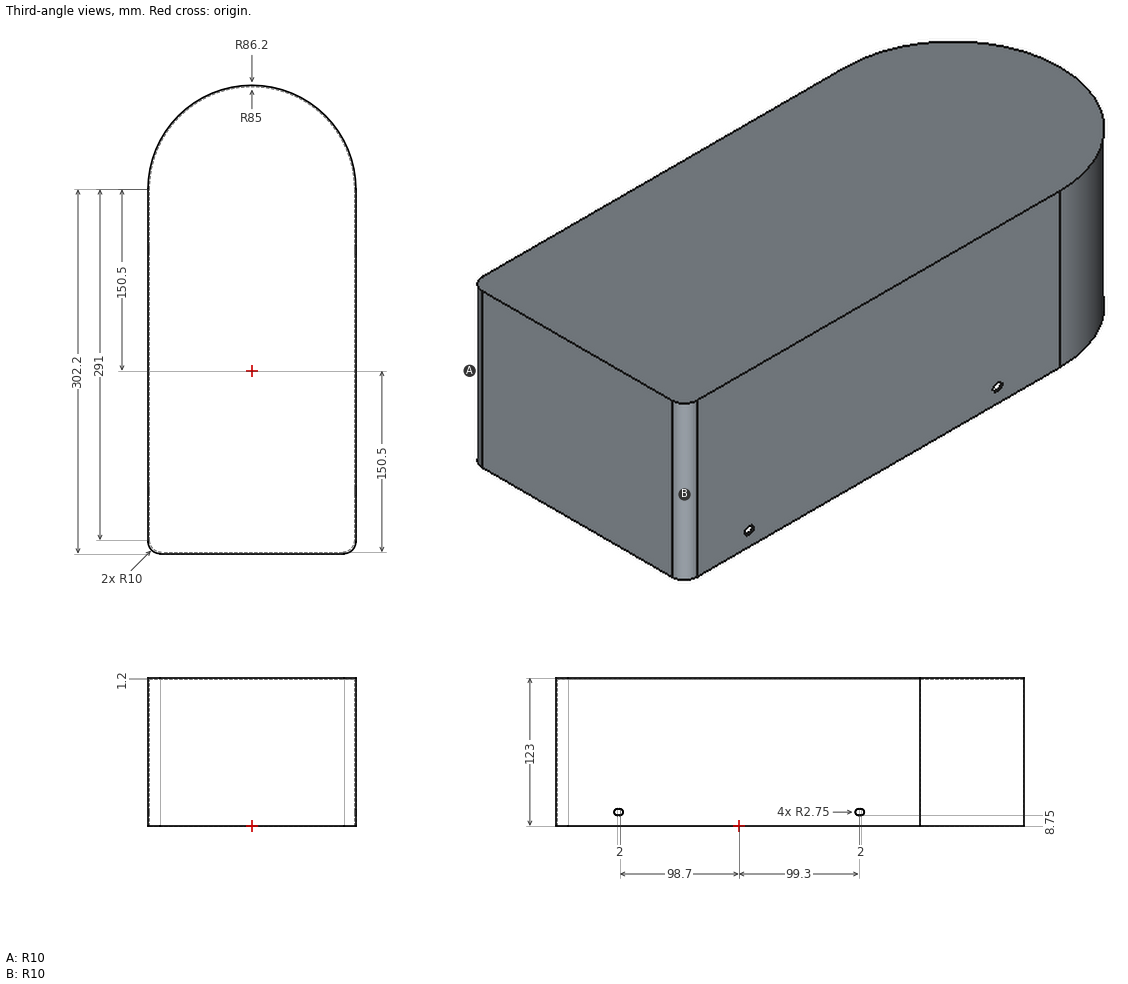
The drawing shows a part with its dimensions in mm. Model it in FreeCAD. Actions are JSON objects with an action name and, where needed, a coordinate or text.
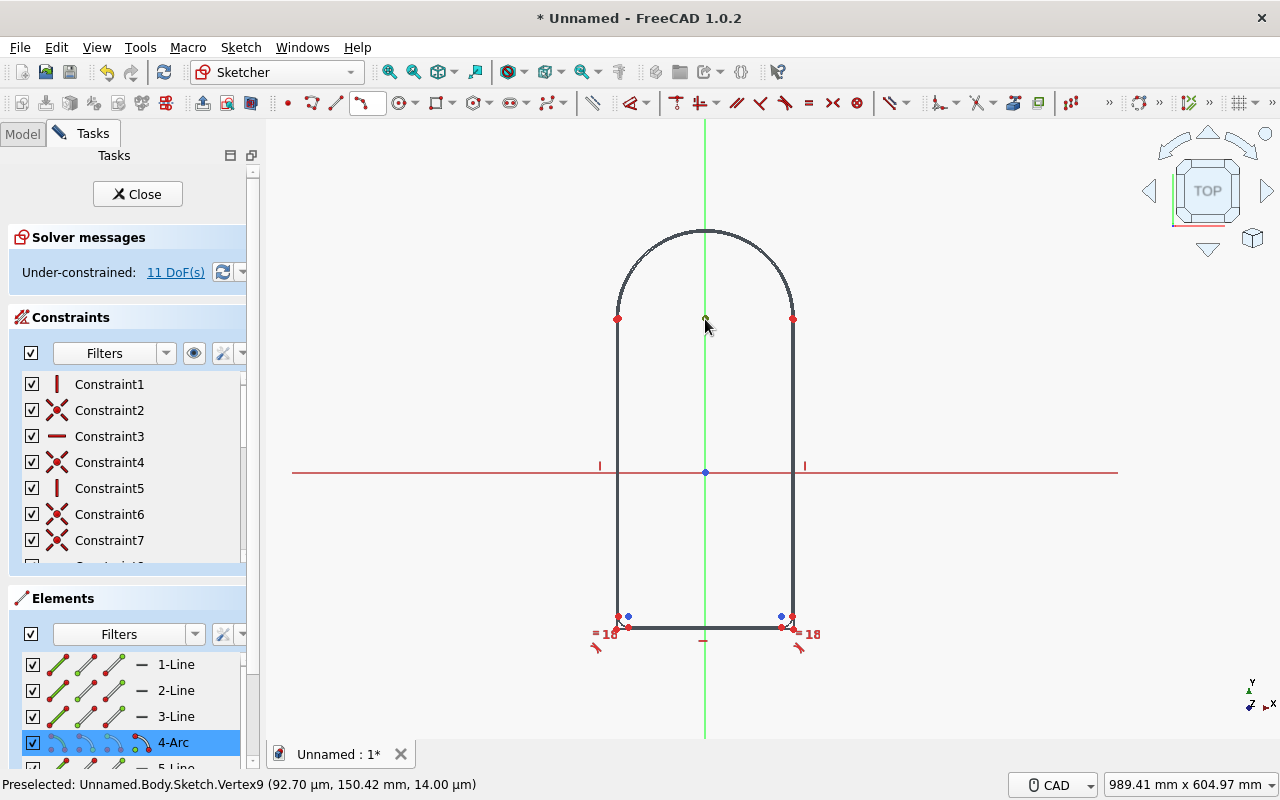
{"action": "left_click", "coordinate": [705, 671]}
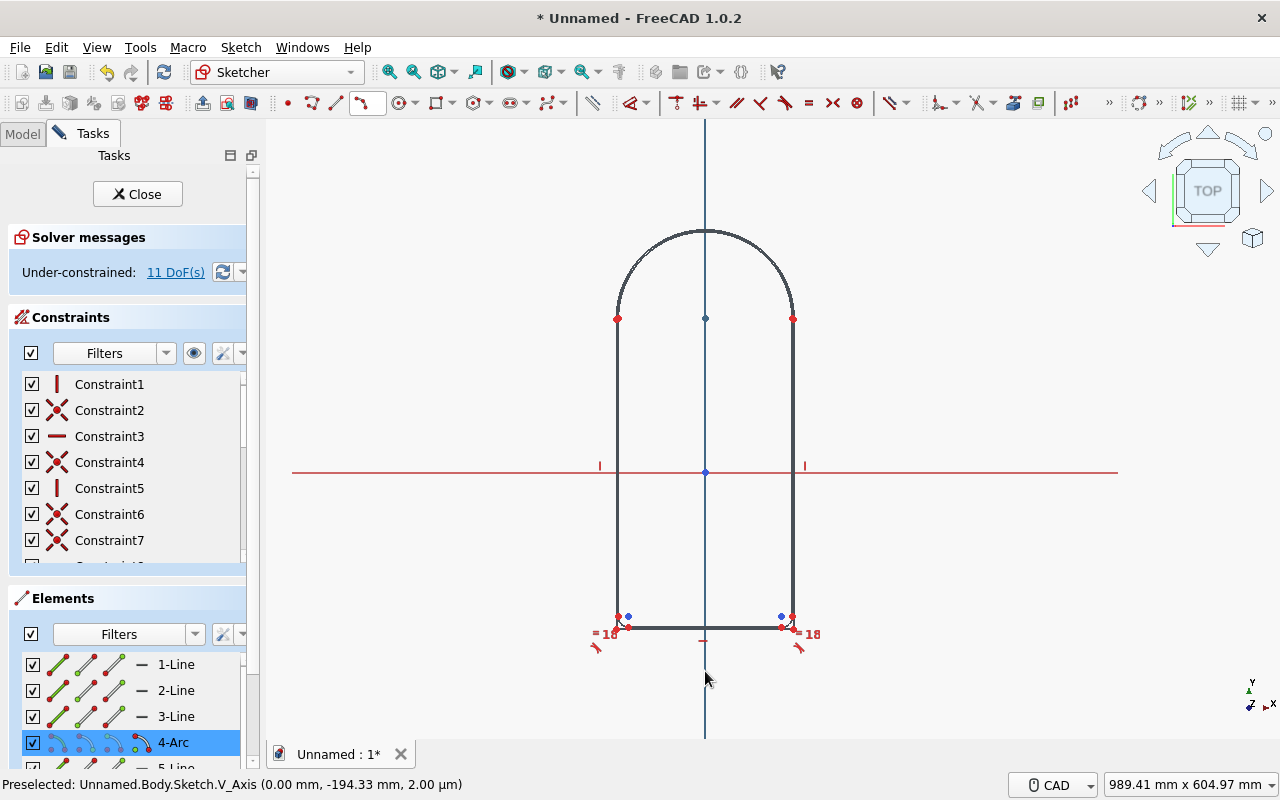
{"action": "key", "text": "c"}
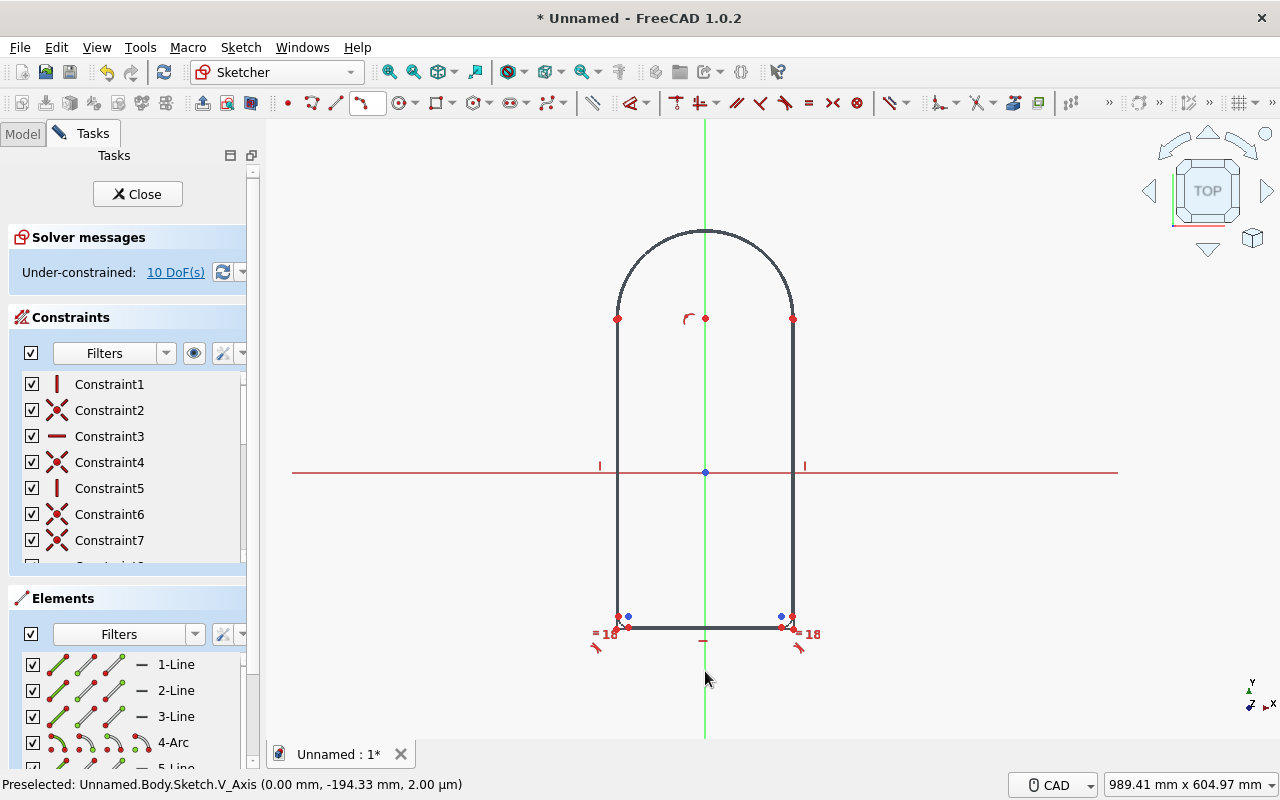
{"action": "left_click", "coordinate": [630, 104]}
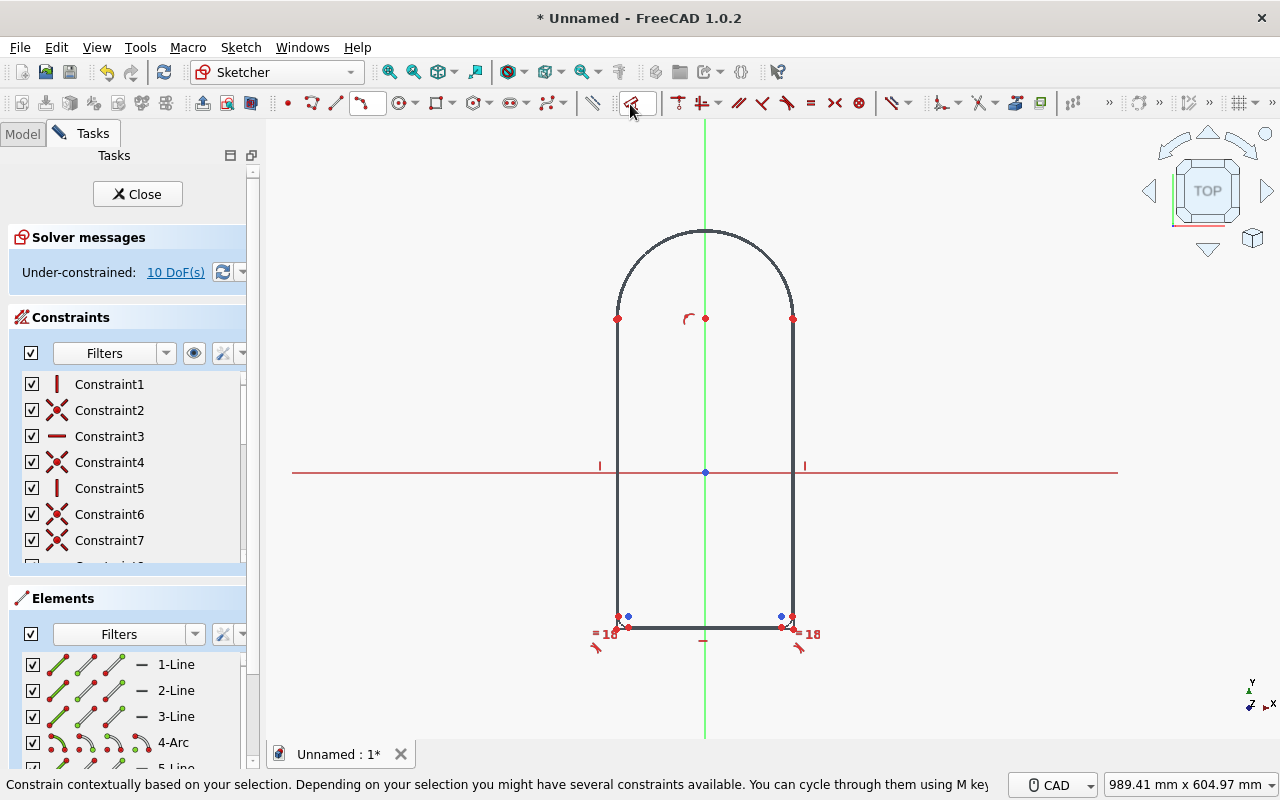
{"action": "scroll", "coordinate": [653, 247], "scroll_direction": "up", "scroll_amount": 12}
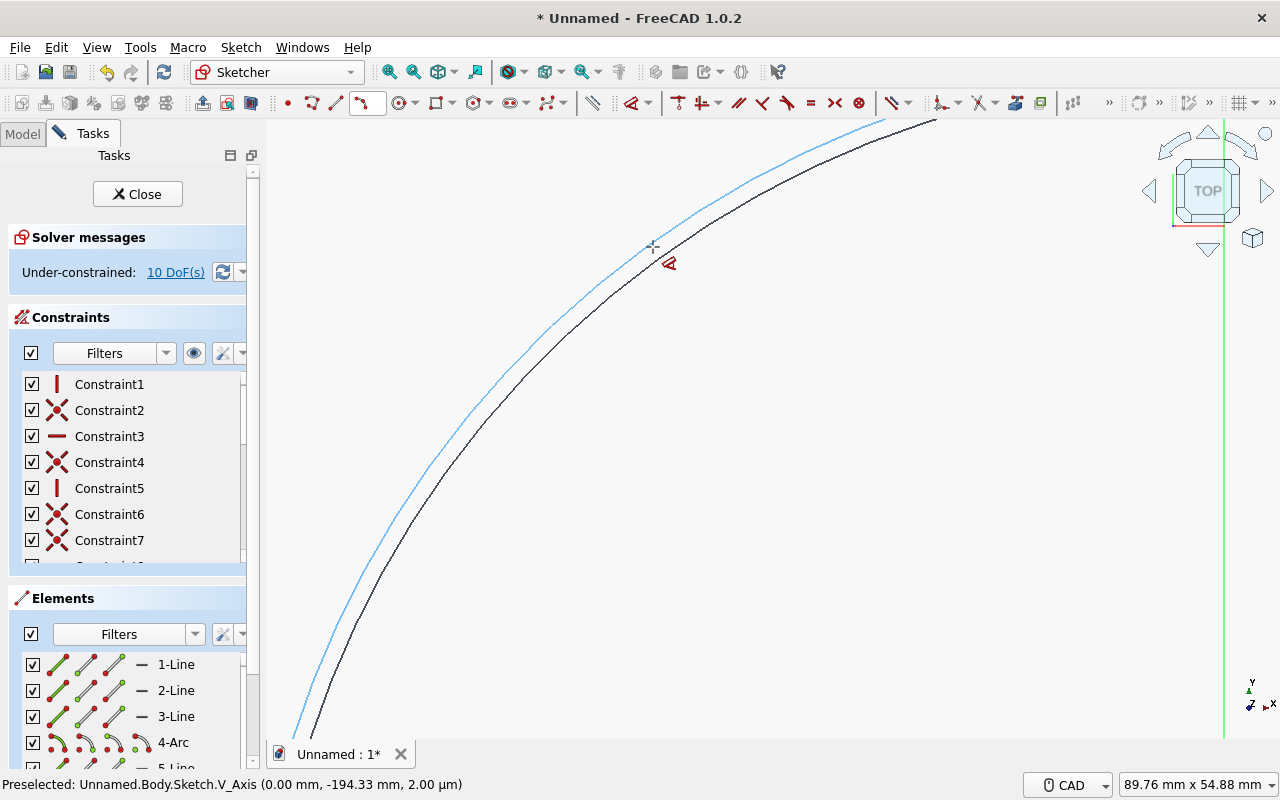
{"action": "left_click", "coordinate": [647, 247]}
{"action": "left_click", "coordinate": [628, 221]}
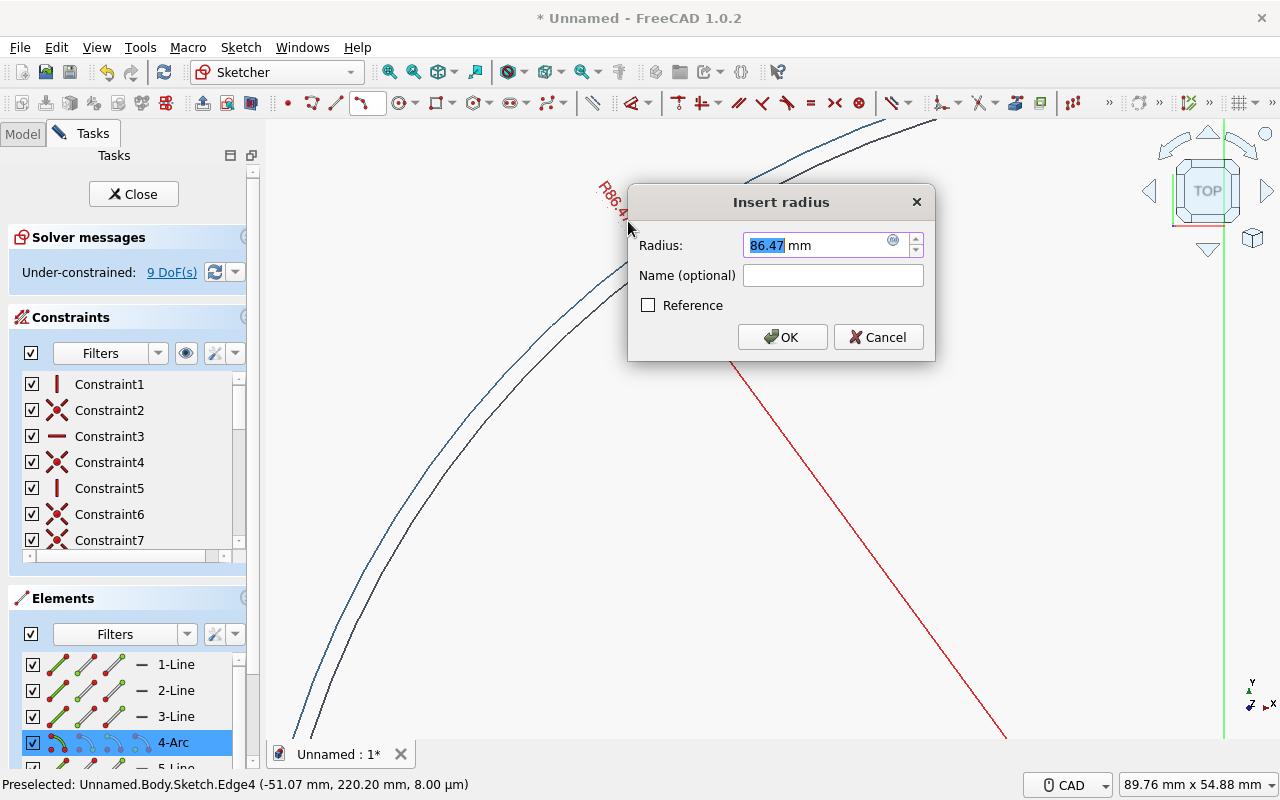
{"action": "type", "text": "86.2"}
{"action": "key", "text": "Return"}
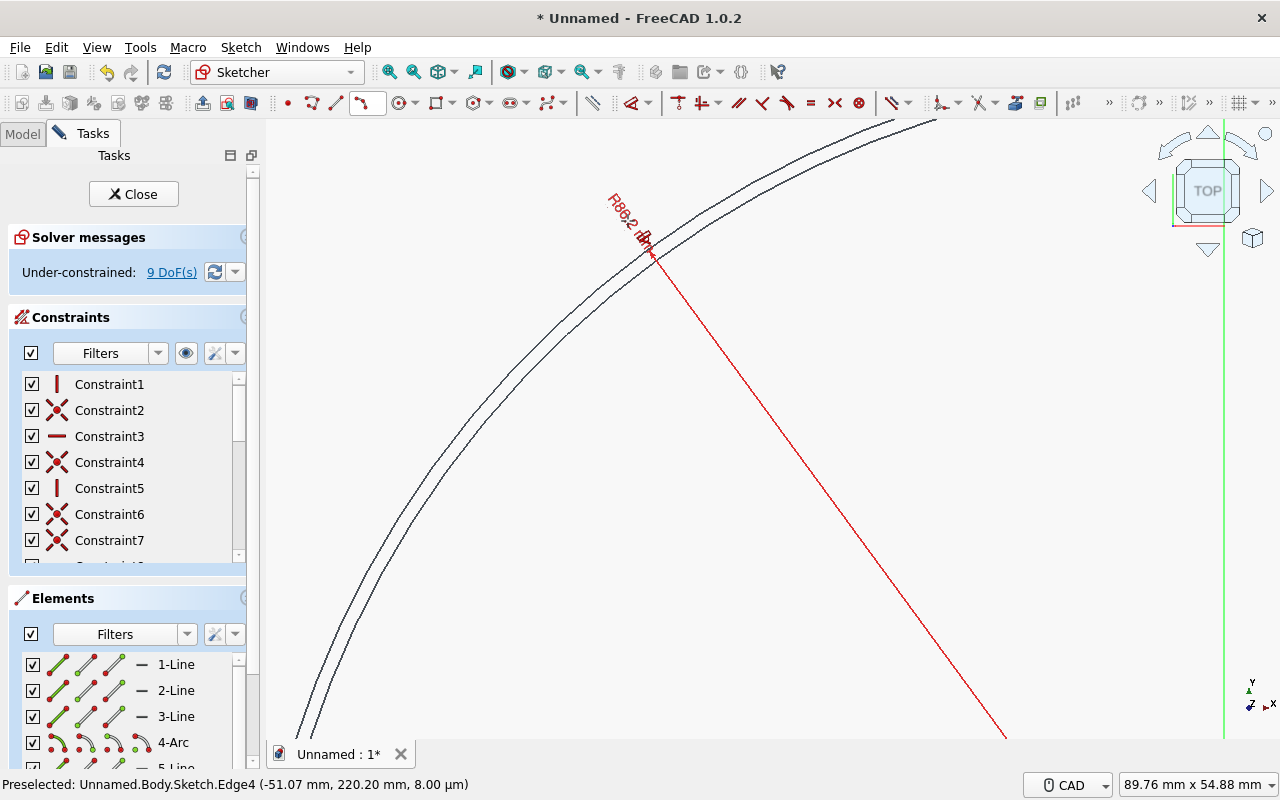
{"action": "scroll", "coordinate": [653, 247], "scroll_direction": "down", "scroll_amount": 12}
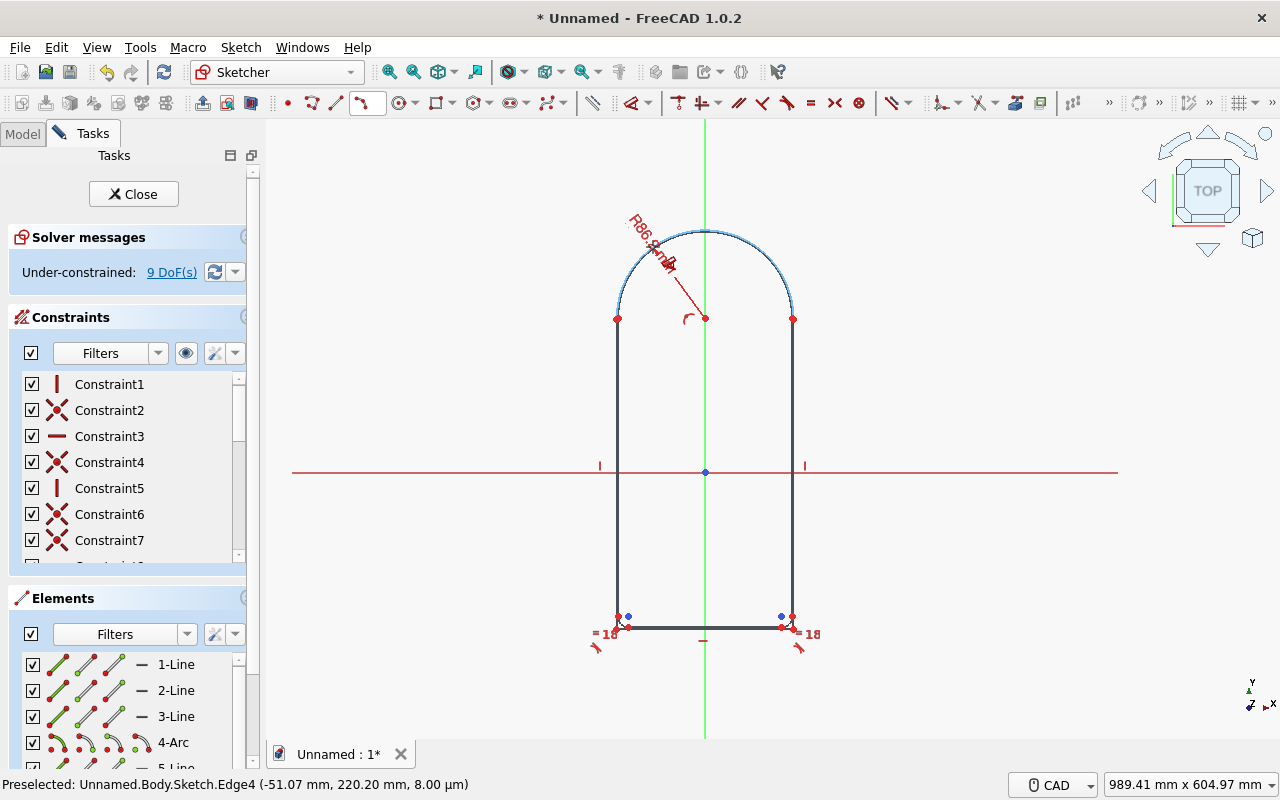
{"action": "scroll", "coordinate": [619, 622], "scroll_direction": "up", "scroll_amount": 9}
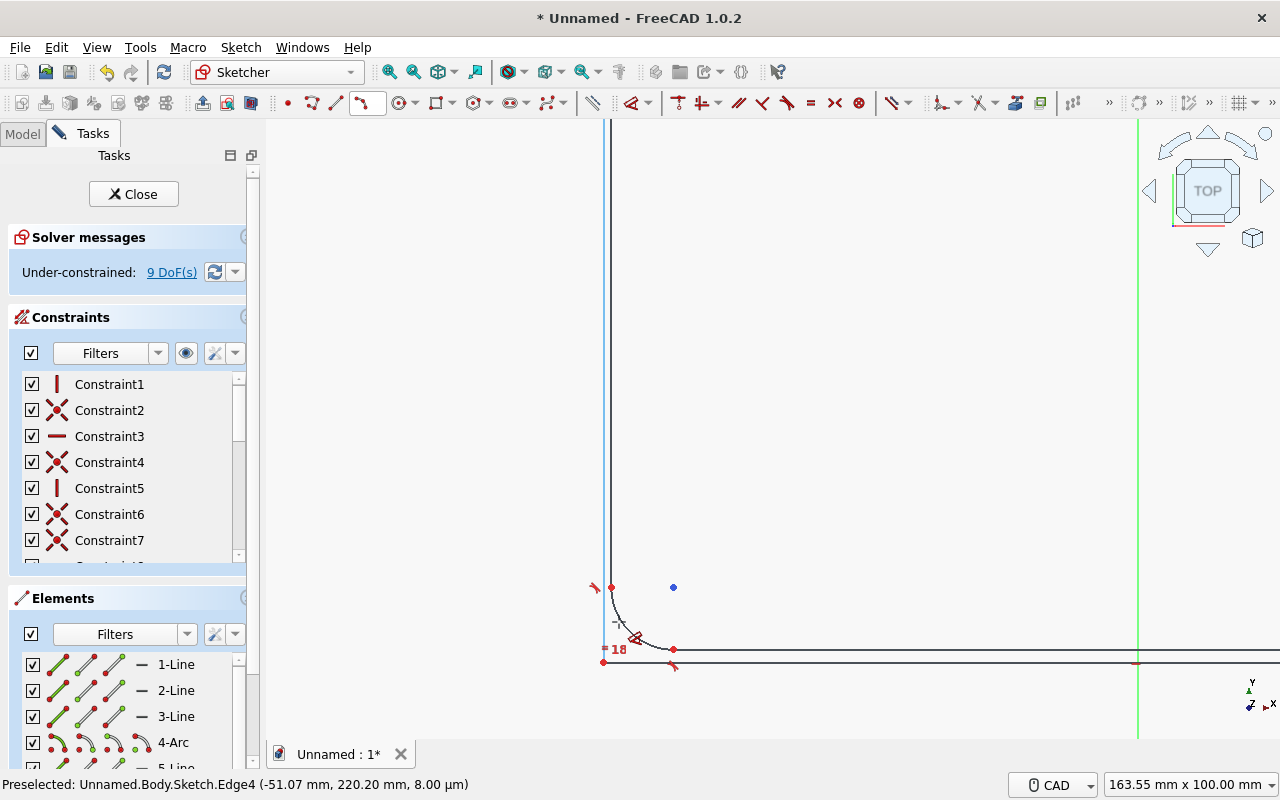
{"action": "left_click", "coordinate": [618, 616]}
{"action": "left_click", "coordinate": [590, 631]}